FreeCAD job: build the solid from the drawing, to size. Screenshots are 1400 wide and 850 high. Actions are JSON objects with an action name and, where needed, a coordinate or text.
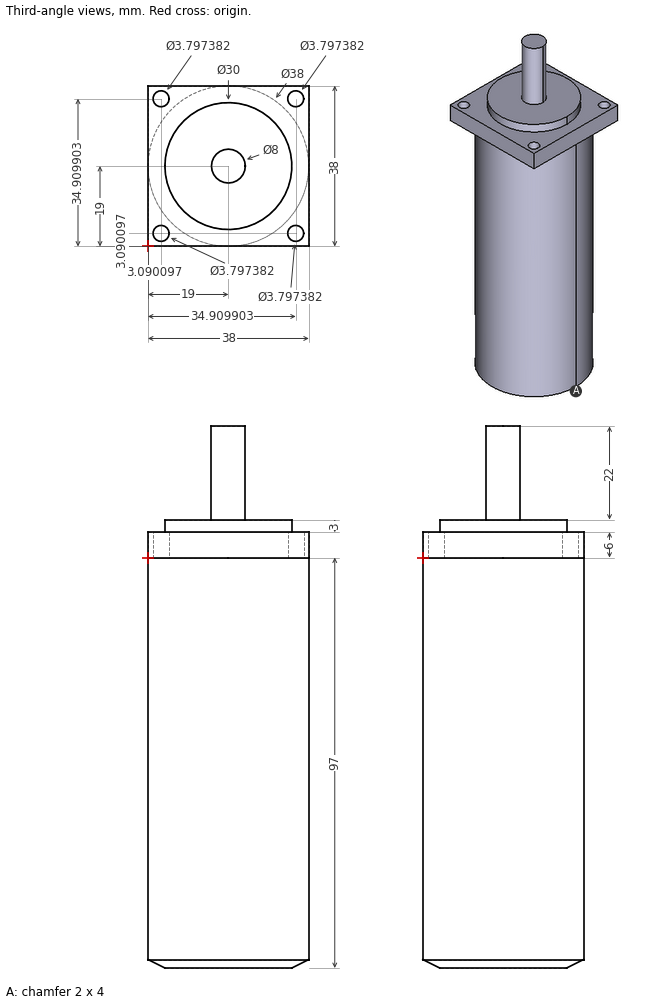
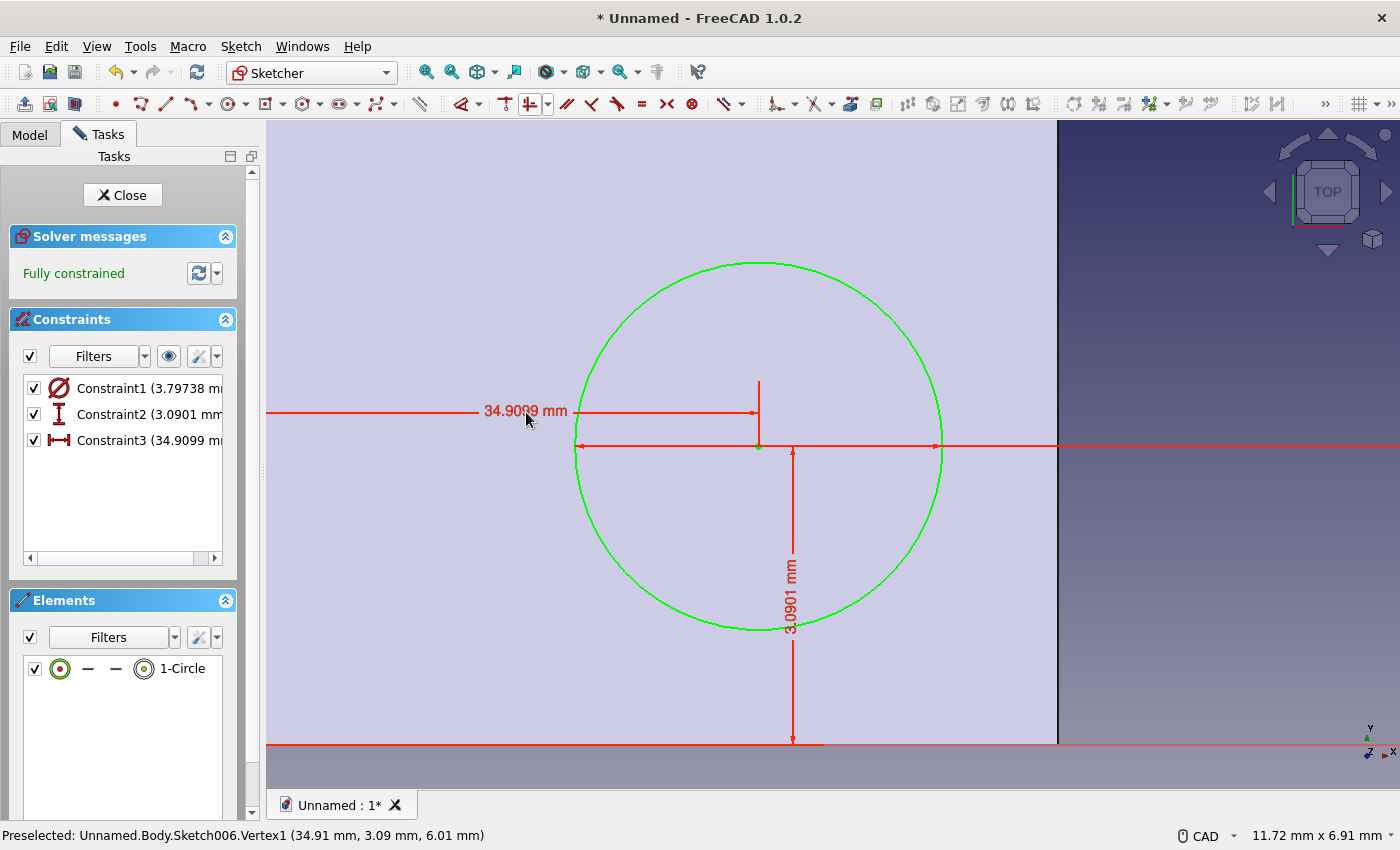
{"action": "left_click", "coordinate": [123, 195]}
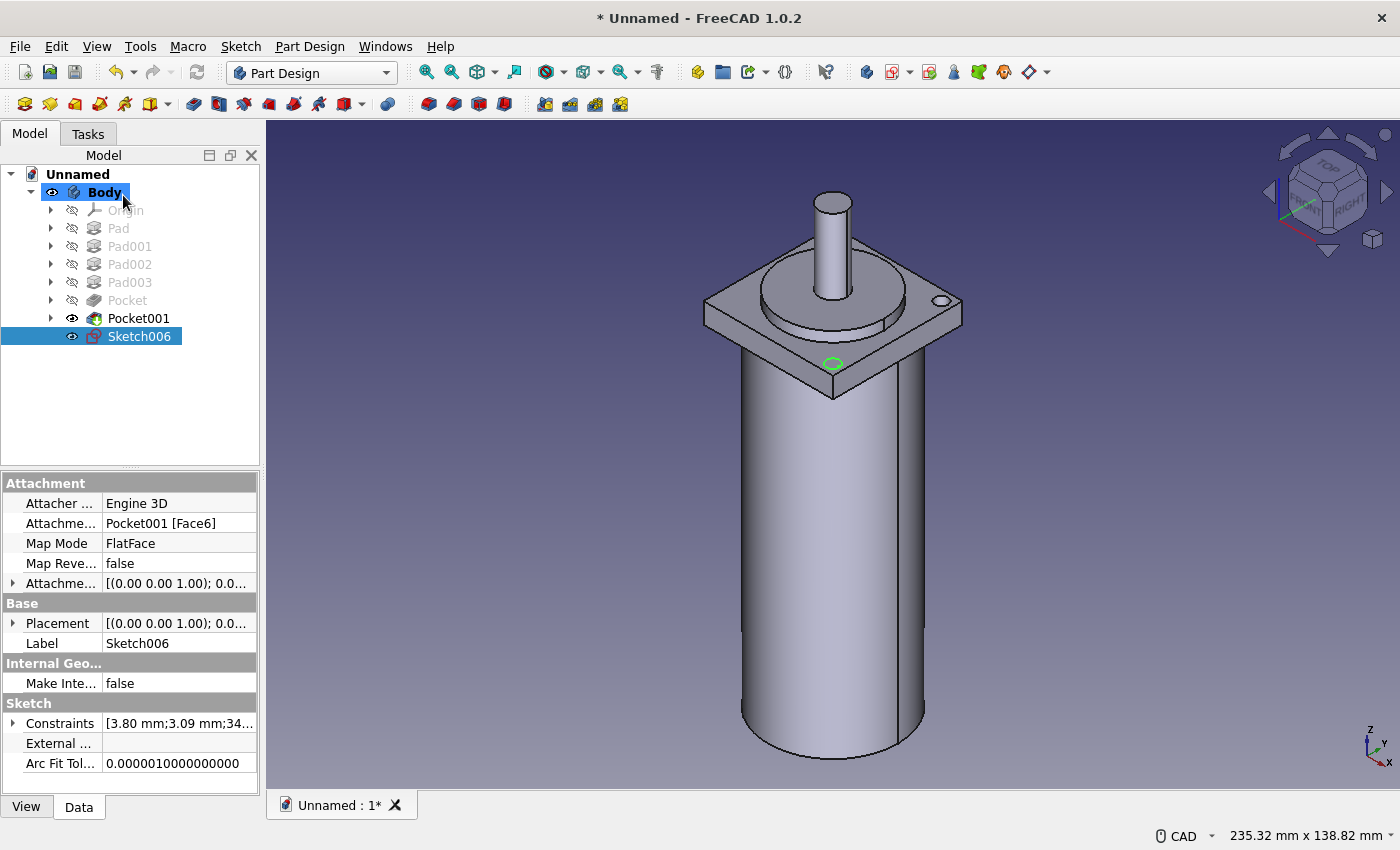
{"action": "left_click", "coordinate": [194, 104]}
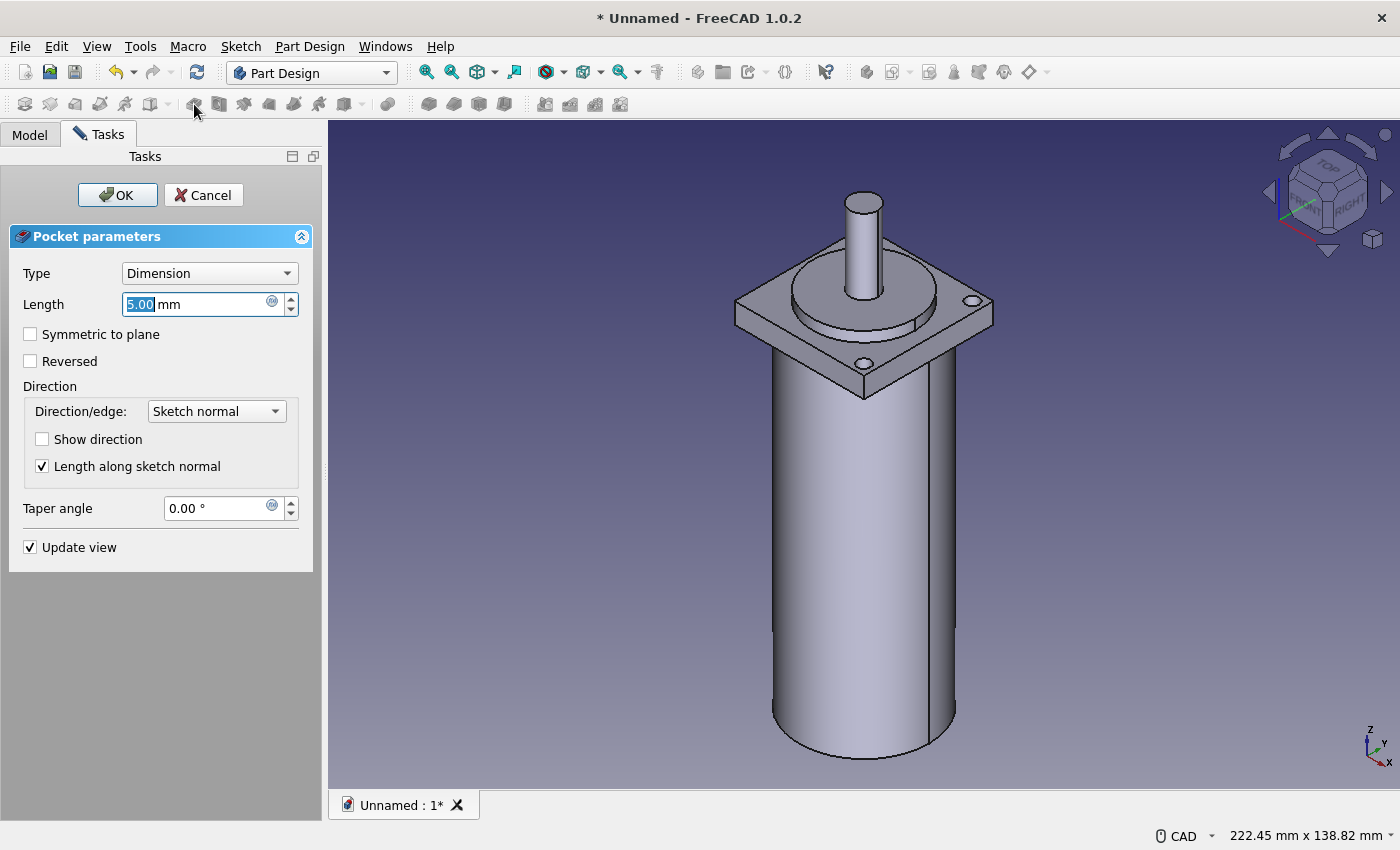
{"action": "left_click", "coordinate": [210, 274]}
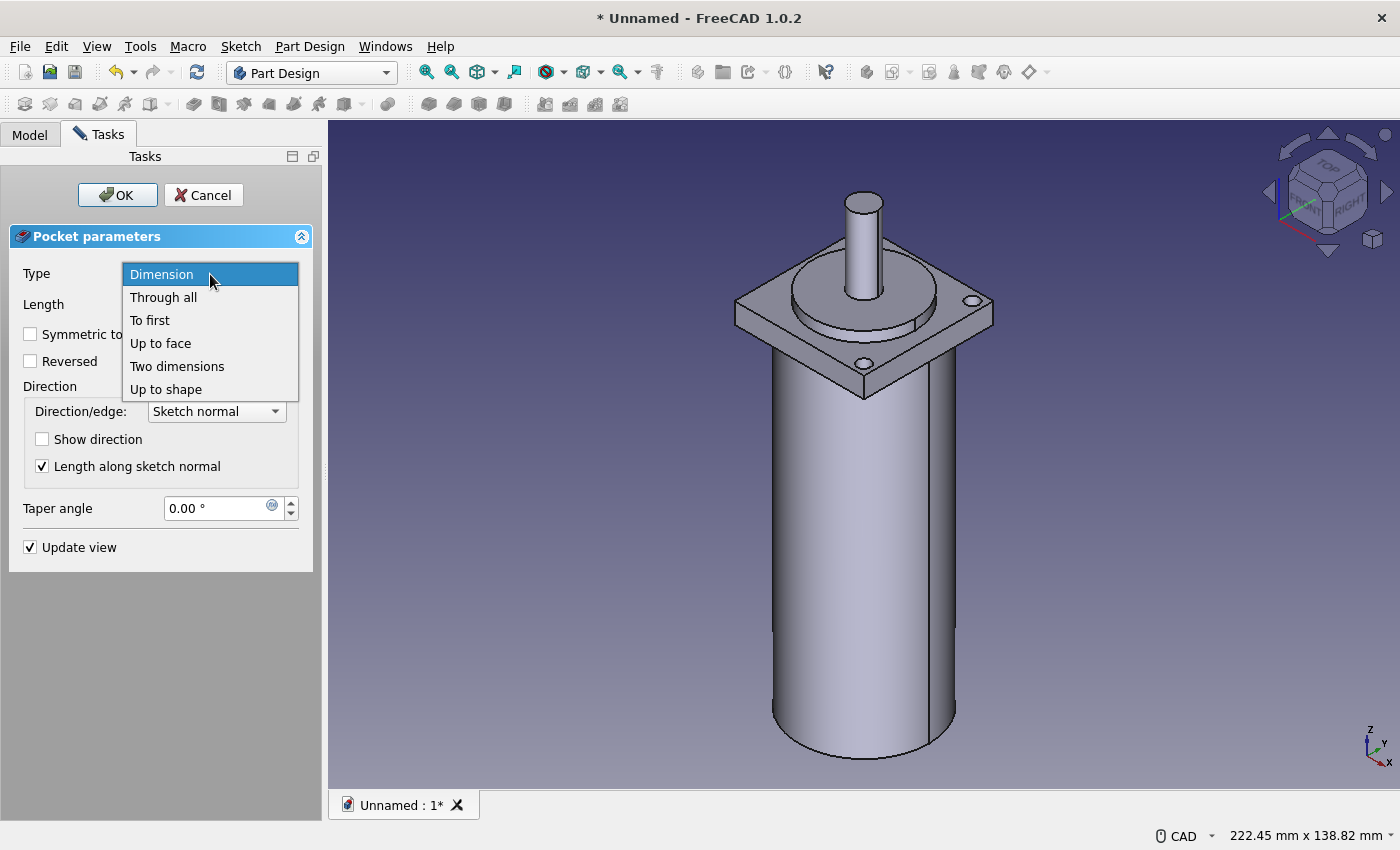
{"action": "left_click", "coordinate": [208, 320]}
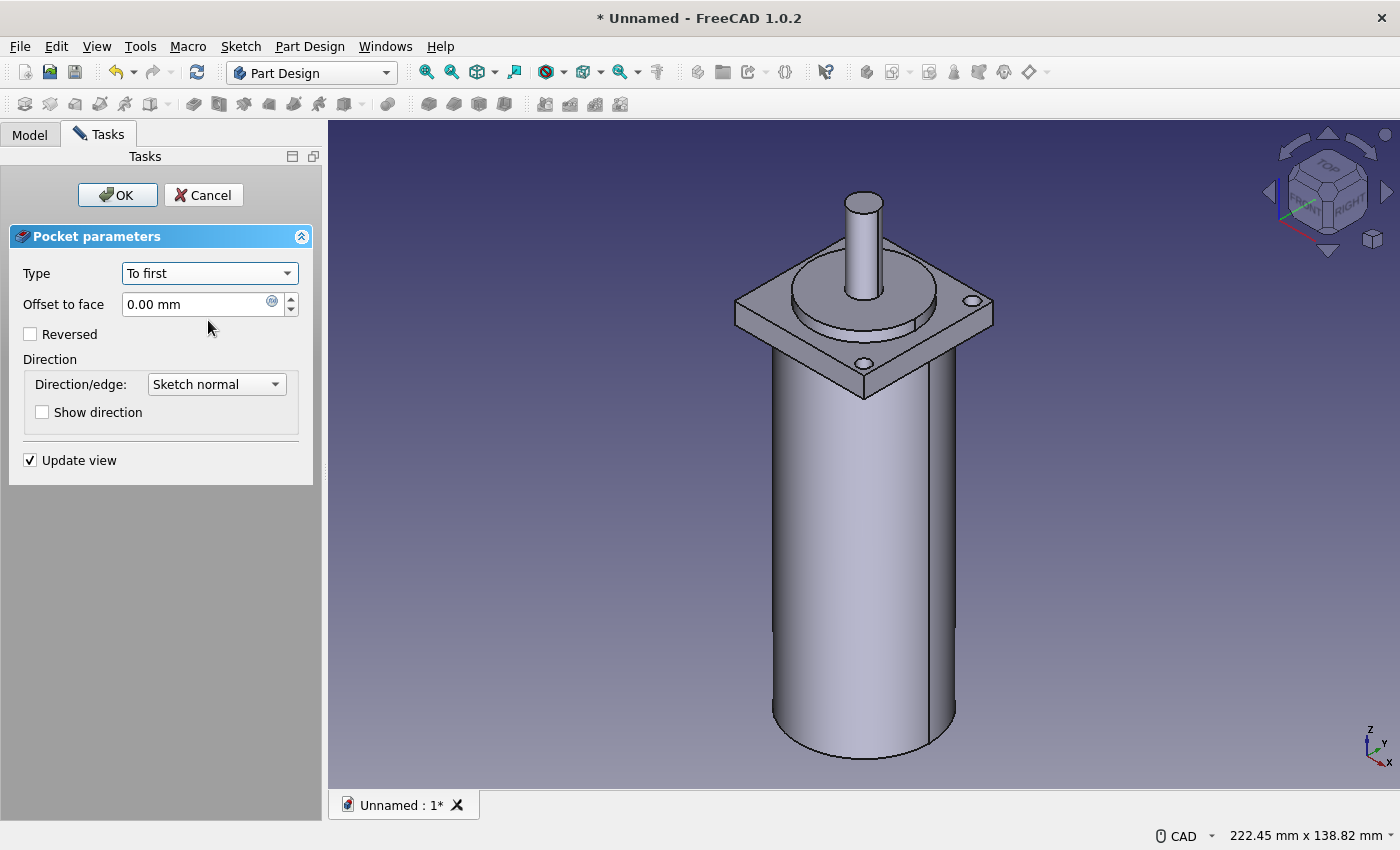
{"action": "left_click", "coordinate": [118, 195]}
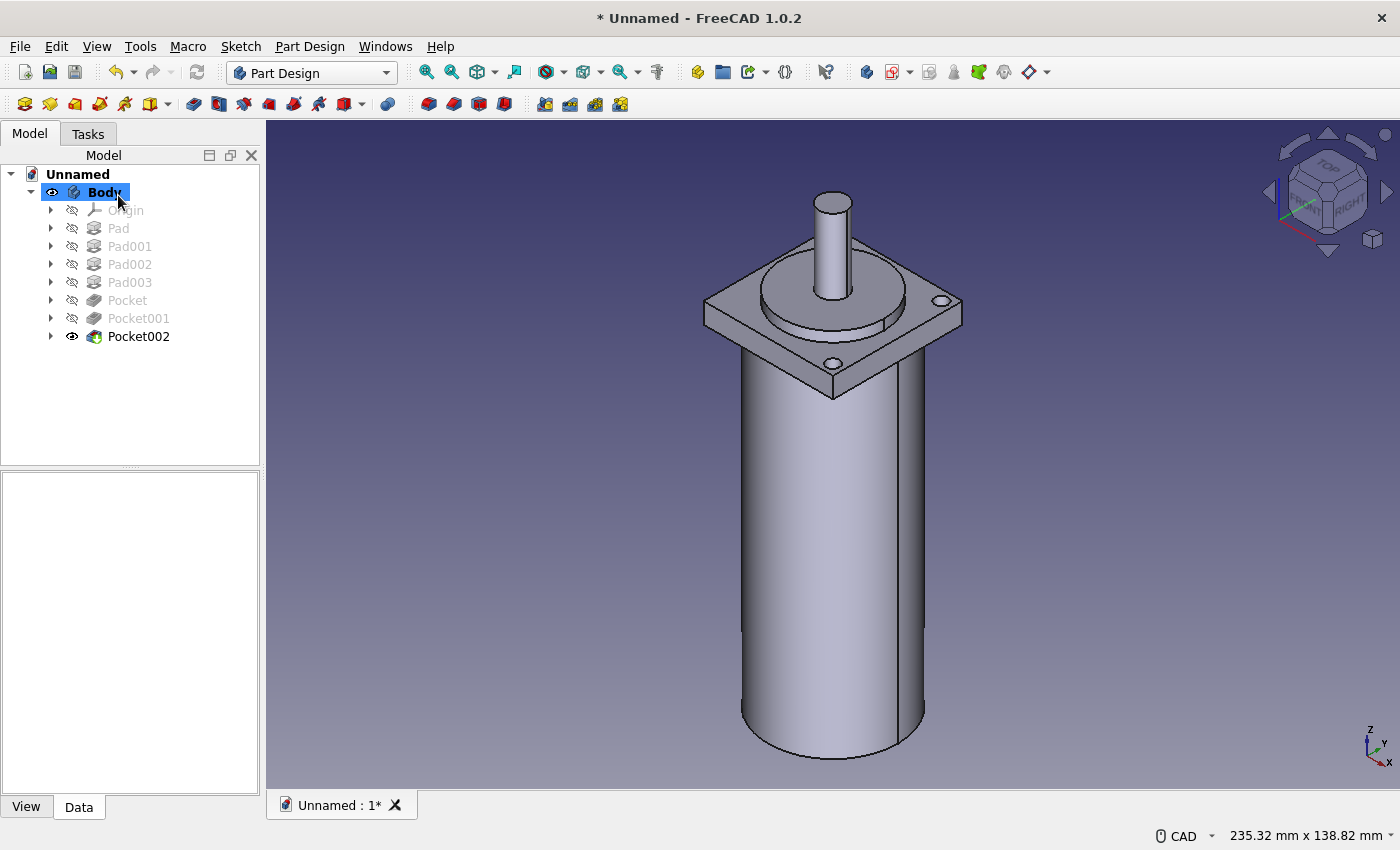
{"action": "left_click", "coordinate": [925, 311]}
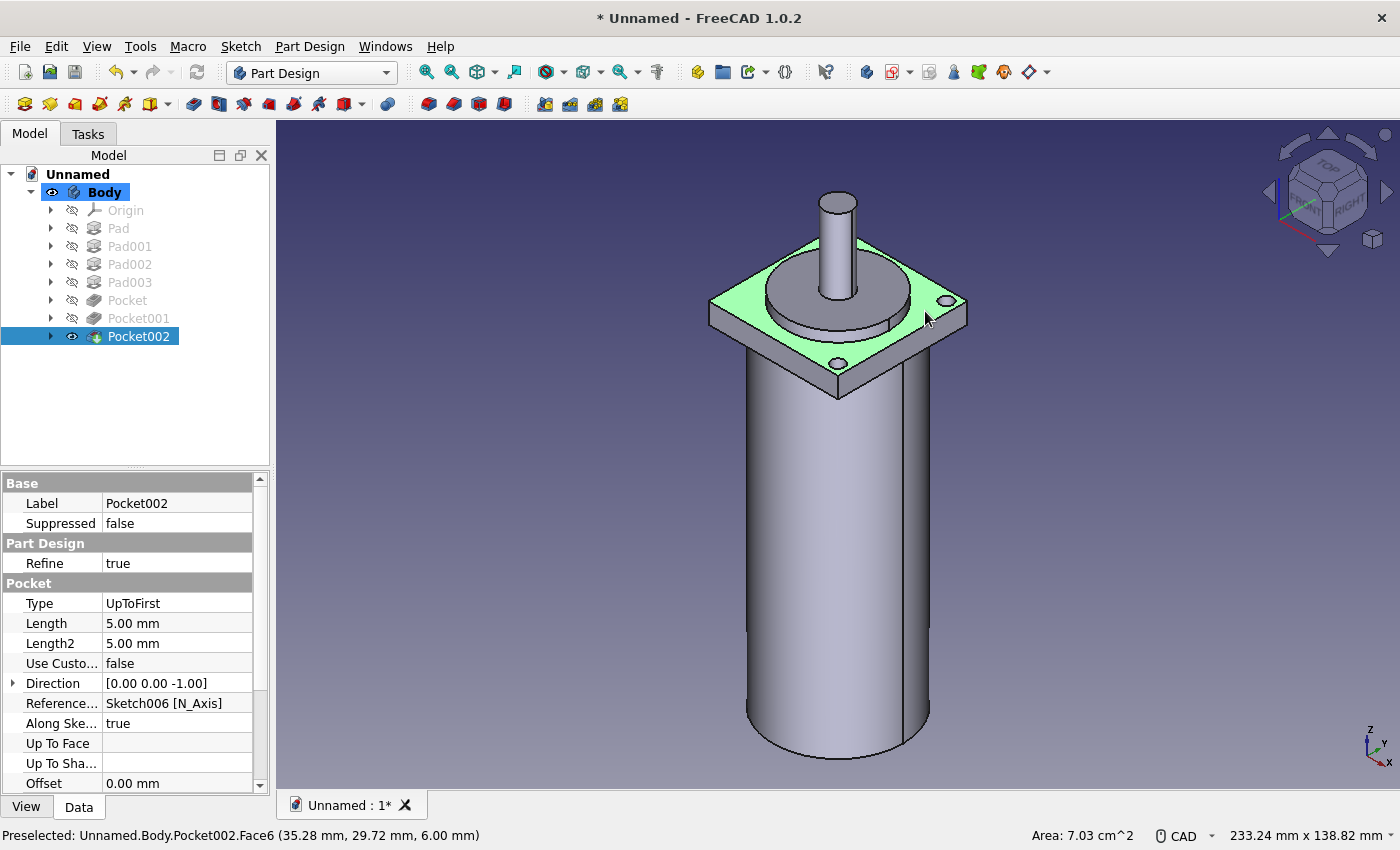
{"action": "left_click", "coordinate": [892, 72]}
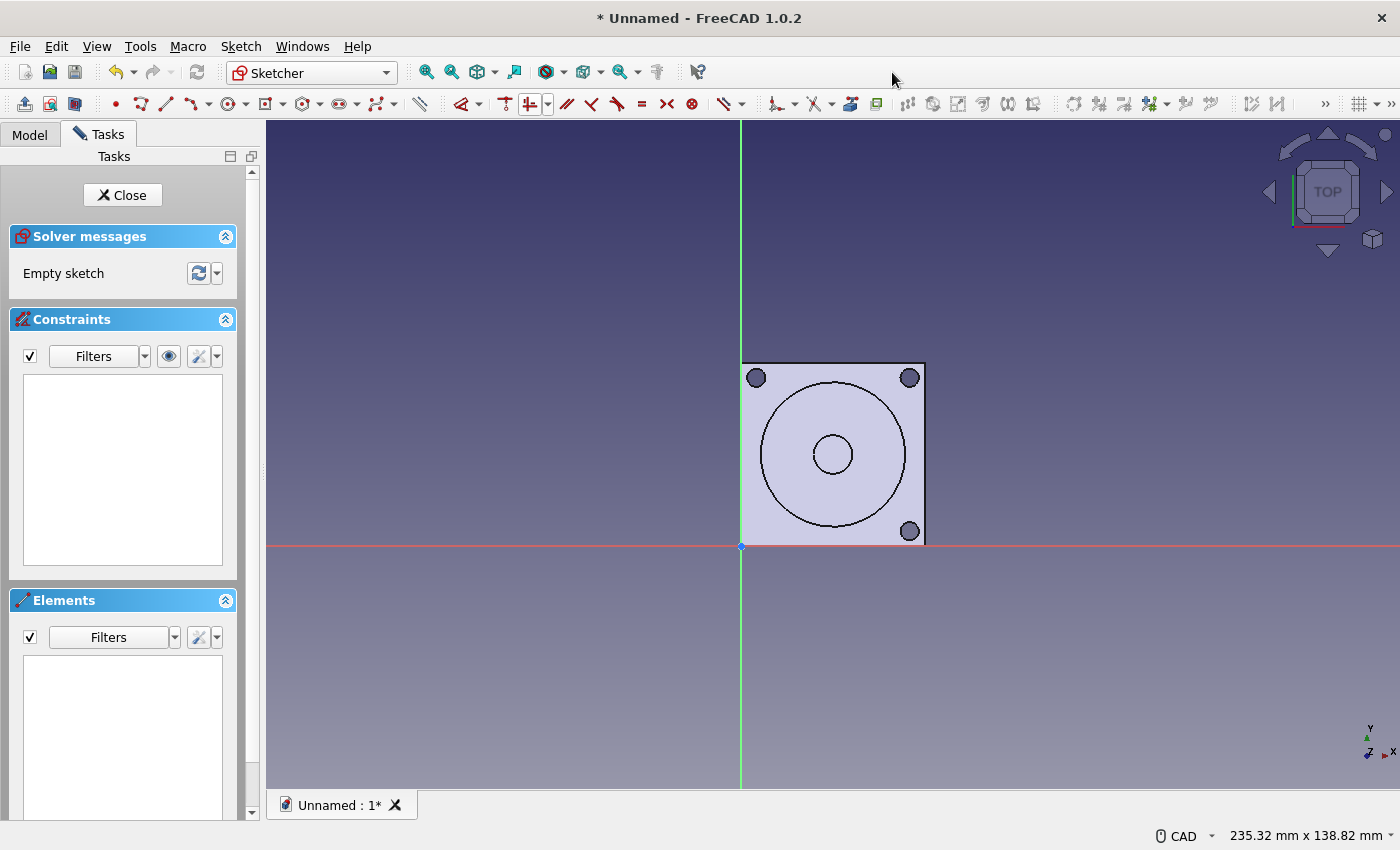
{"action": "scroll", "coordinate": [753, 539], "scroll_direction": "up", "scroll_amount": 14}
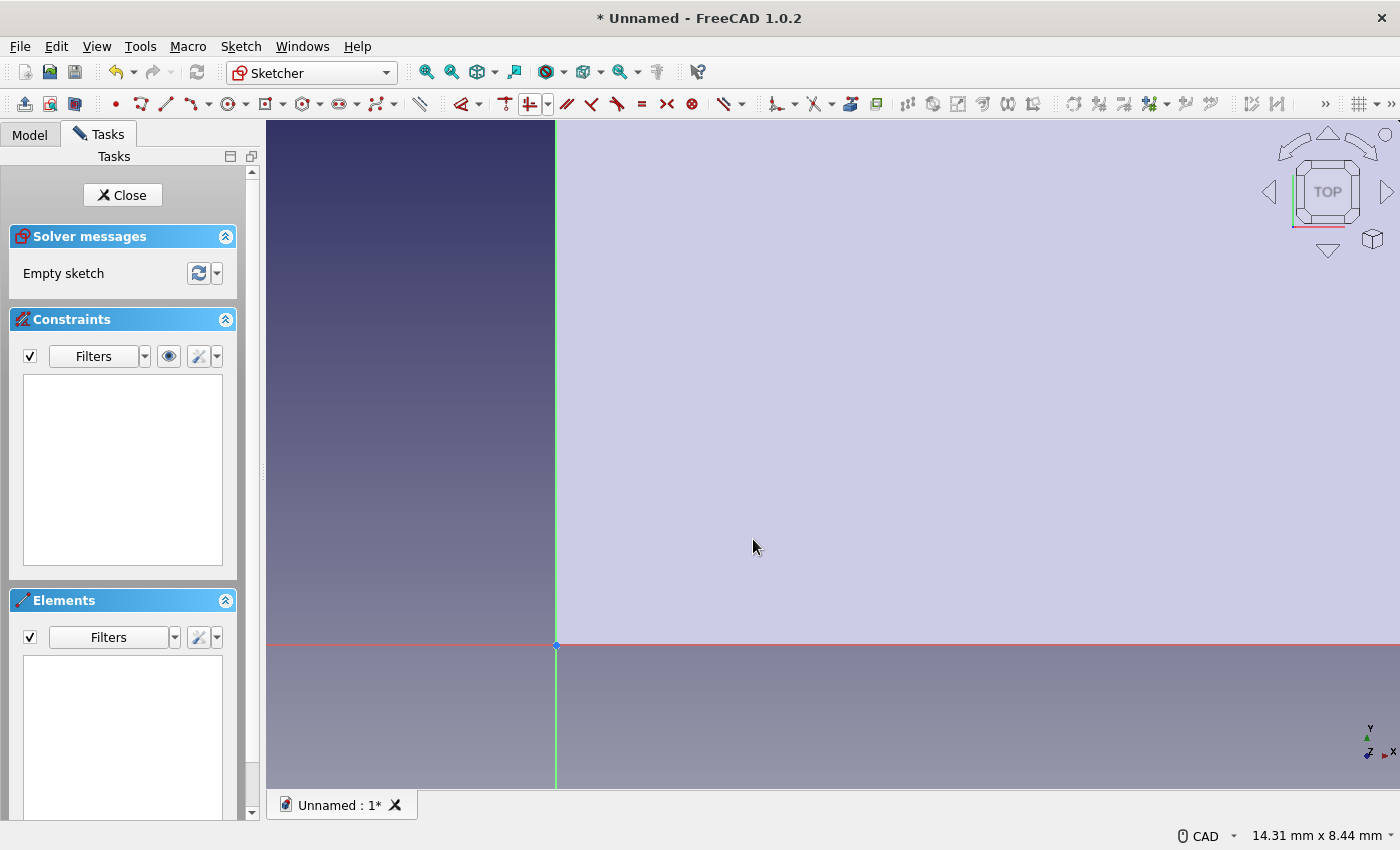
{"action": "left_click", "coordinate": [228, 104]}